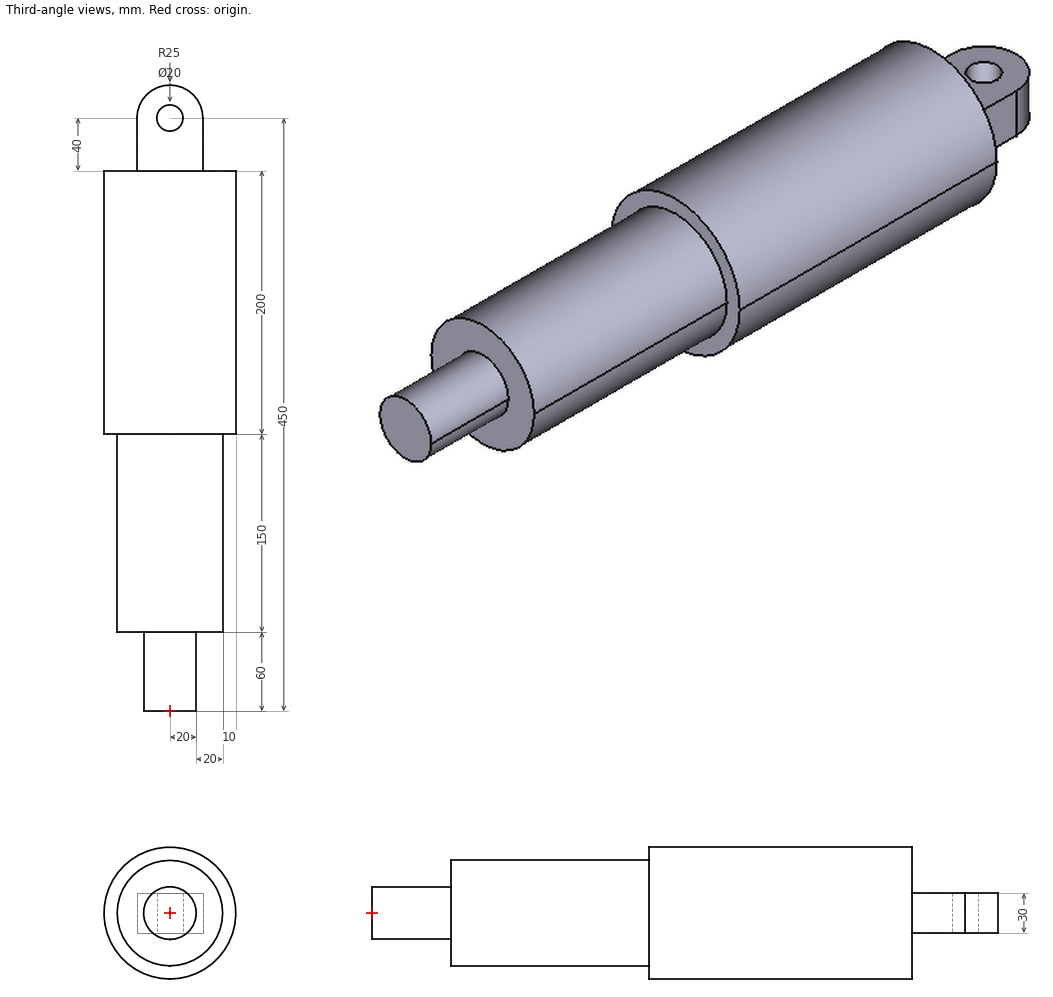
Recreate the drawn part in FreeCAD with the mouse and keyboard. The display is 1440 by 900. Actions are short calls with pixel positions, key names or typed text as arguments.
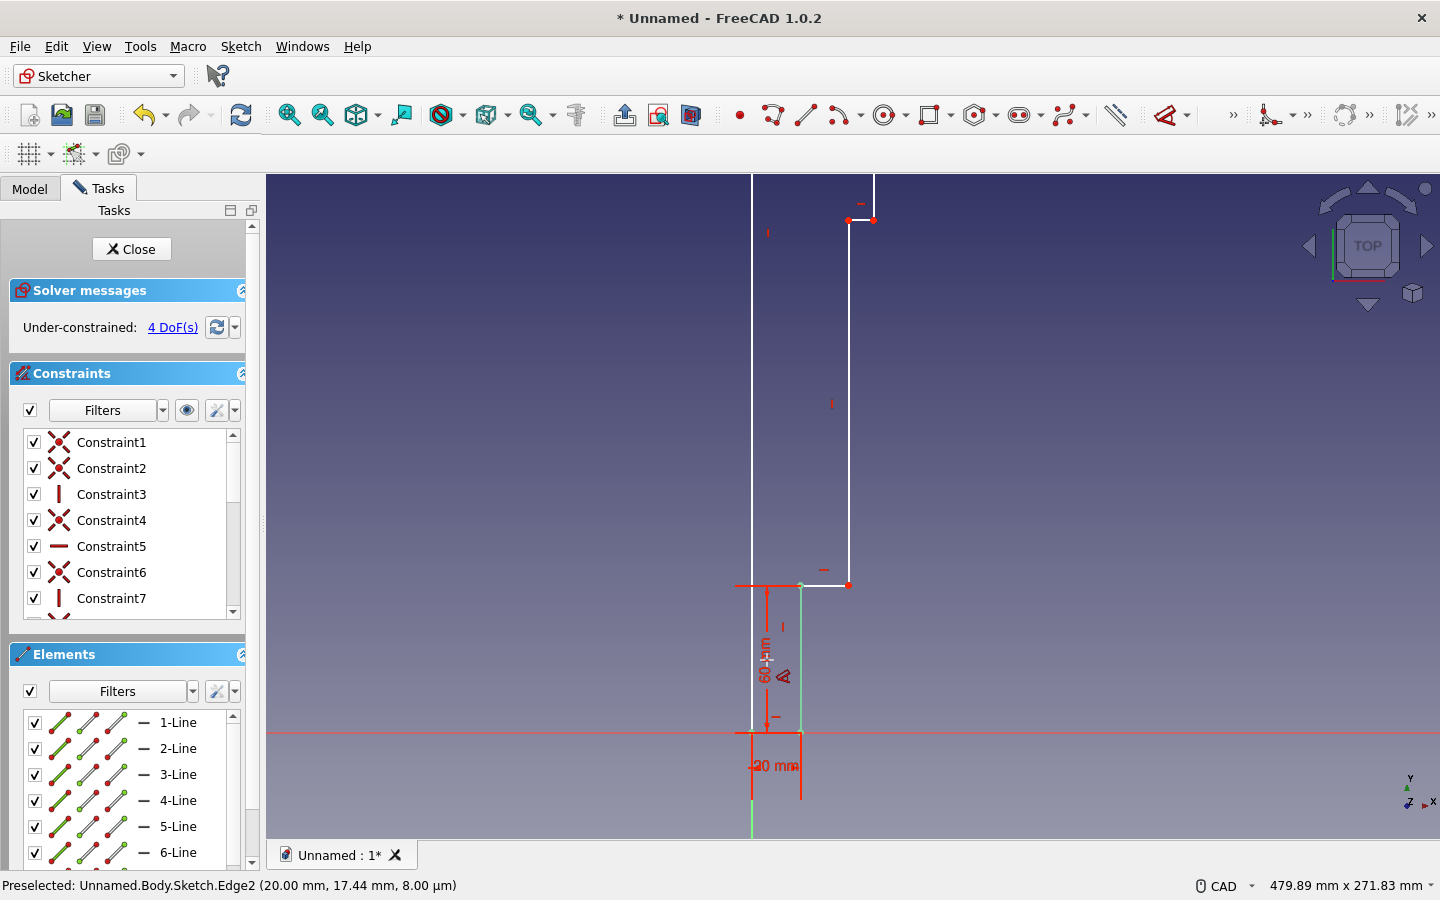
click(815, 586)
click(825, 620)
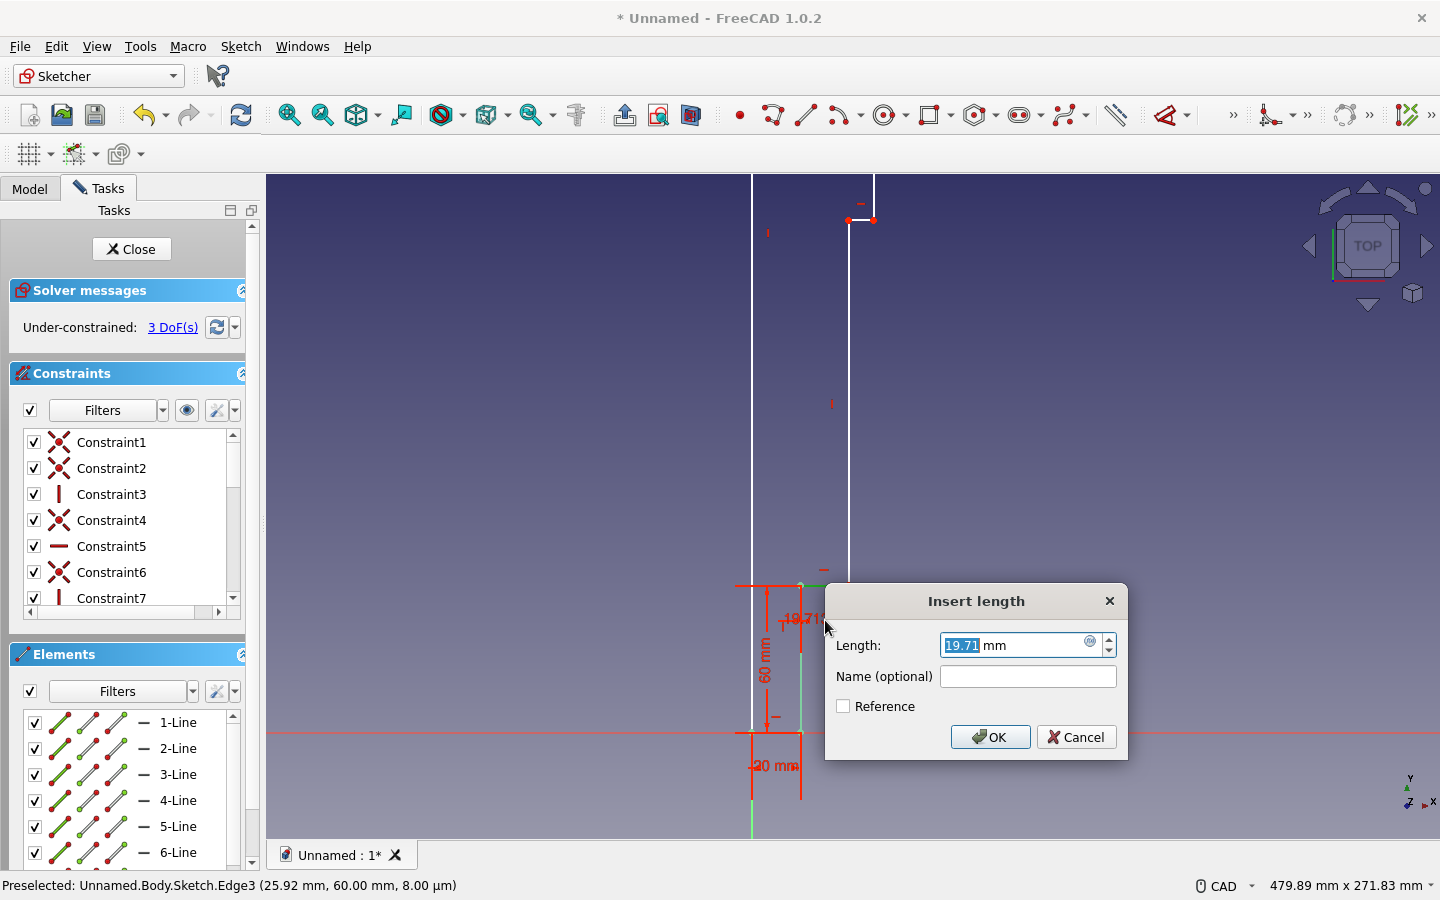
text(20)
key(Return)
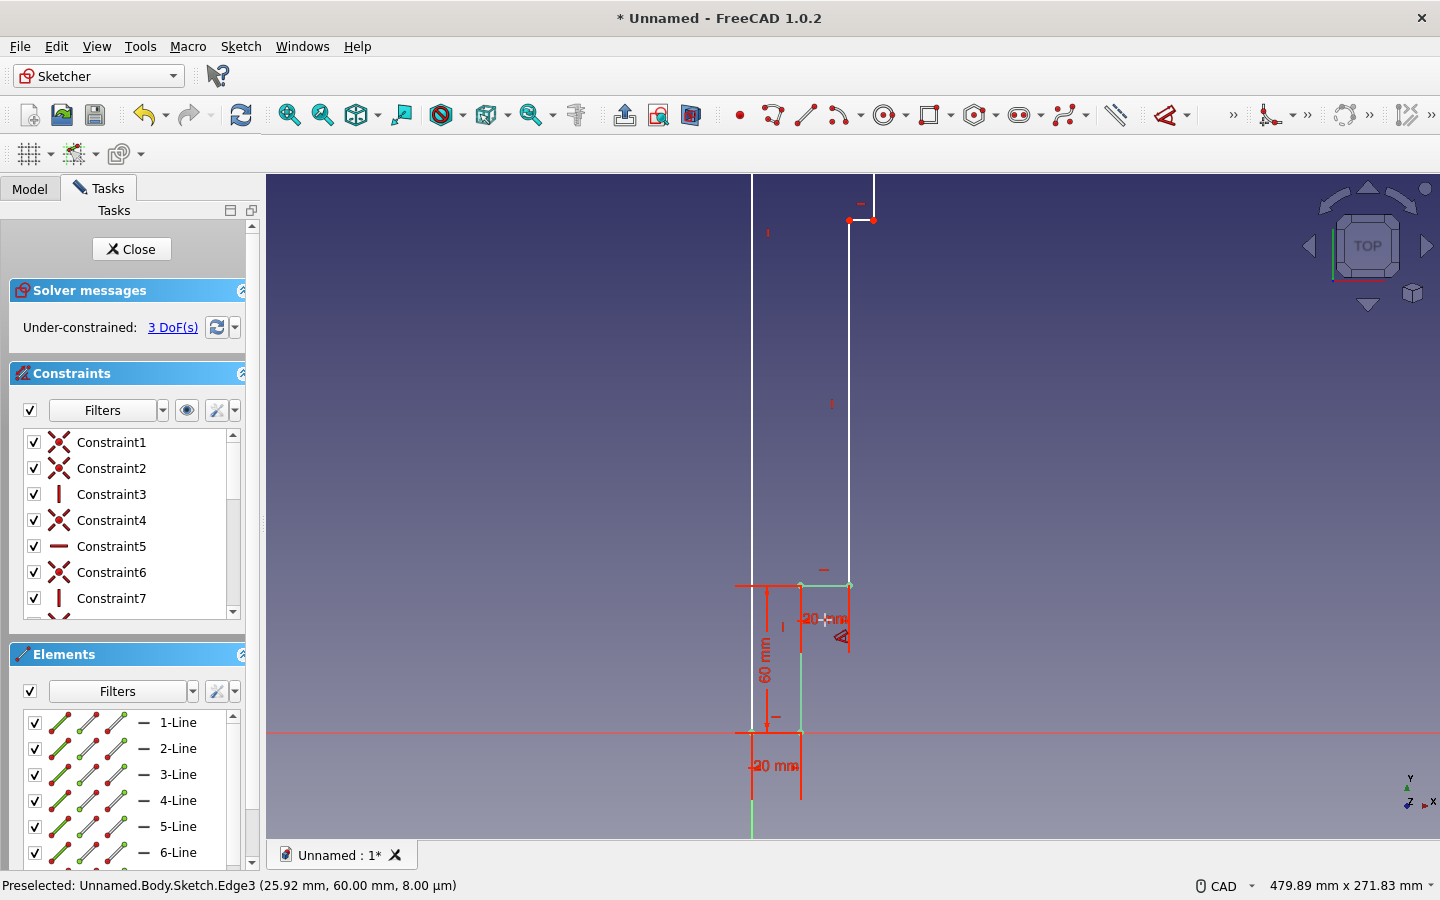
scroll(859, 220, up, 3)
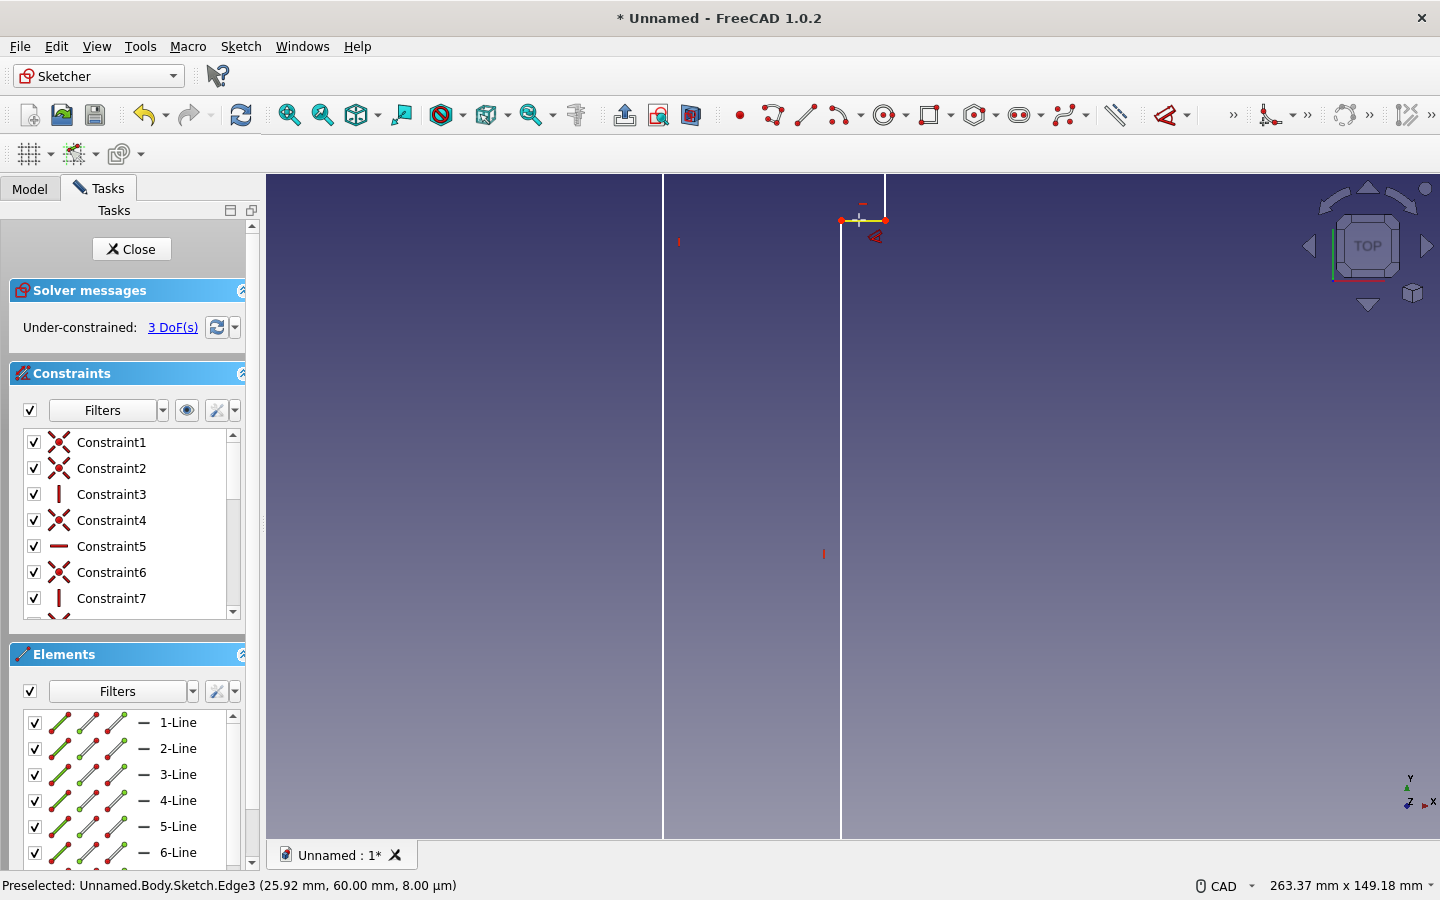
click(859, 221)
click(863, 255)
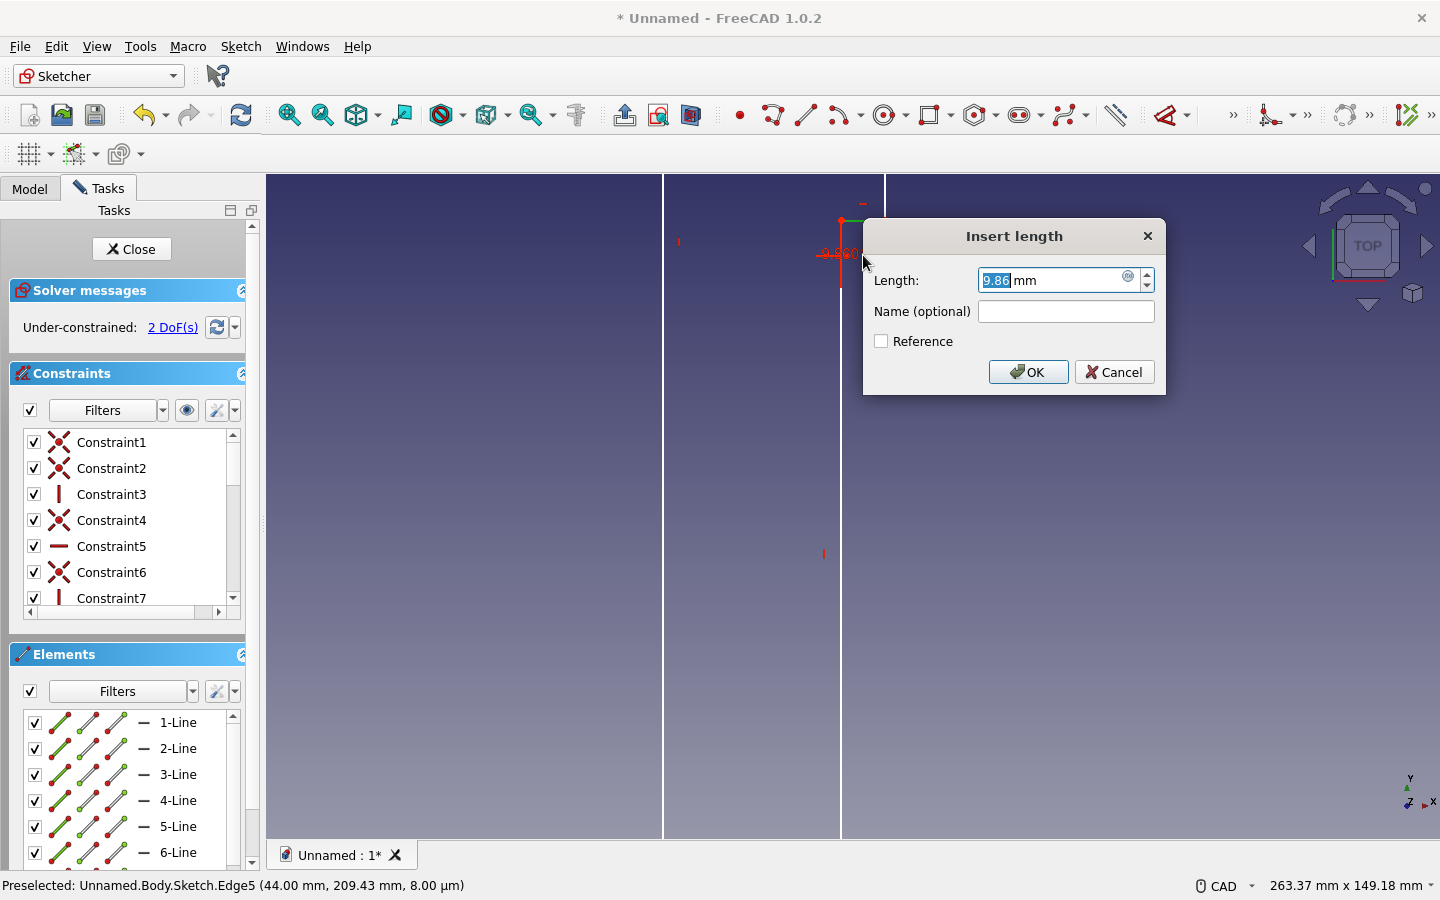
text(10)
key(Return)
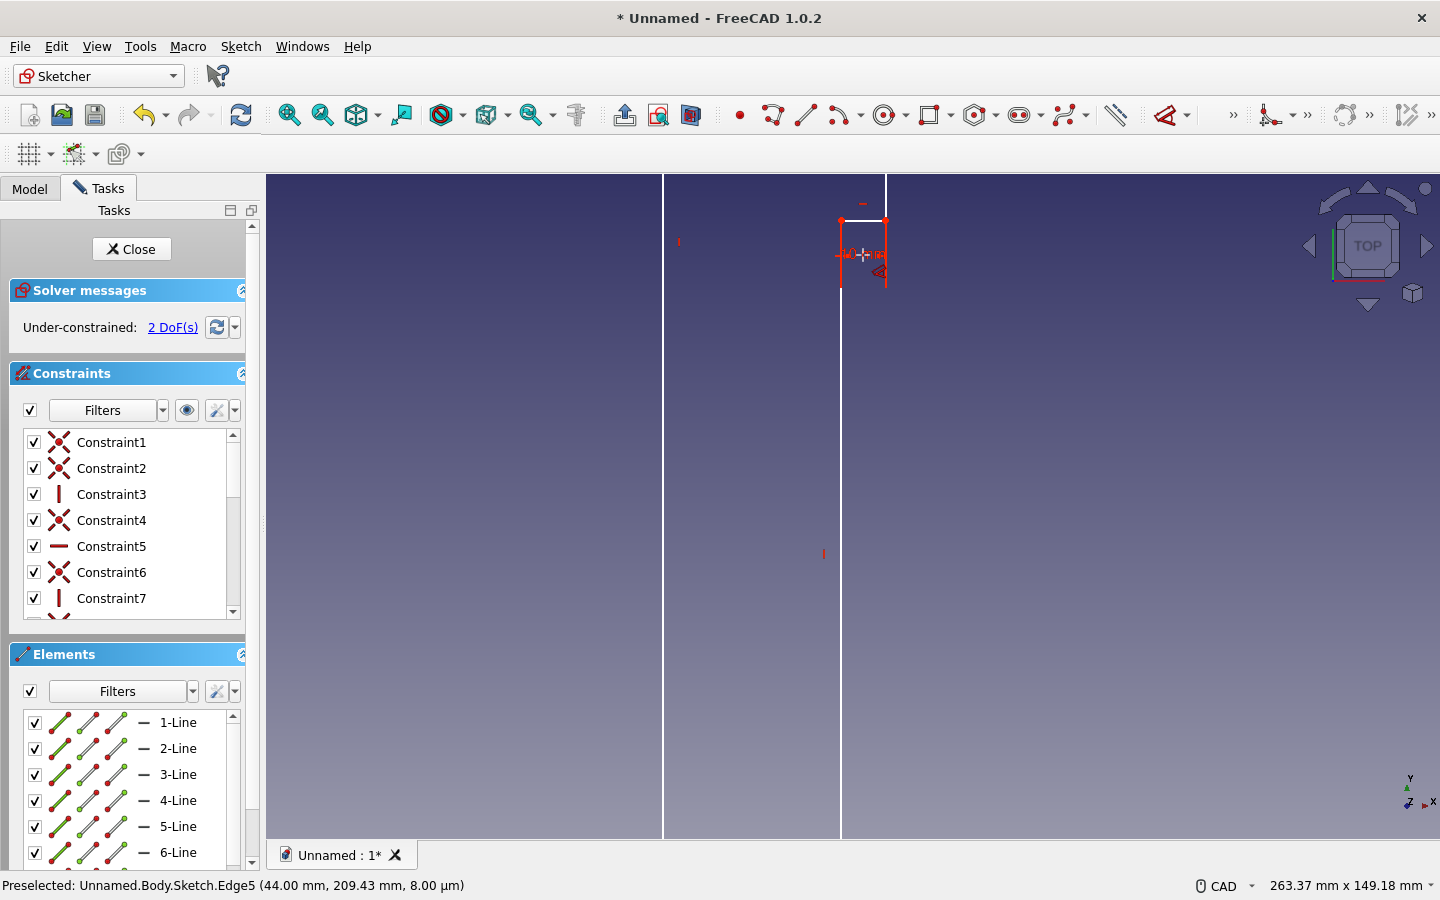
scroll(788, 594, down, 7)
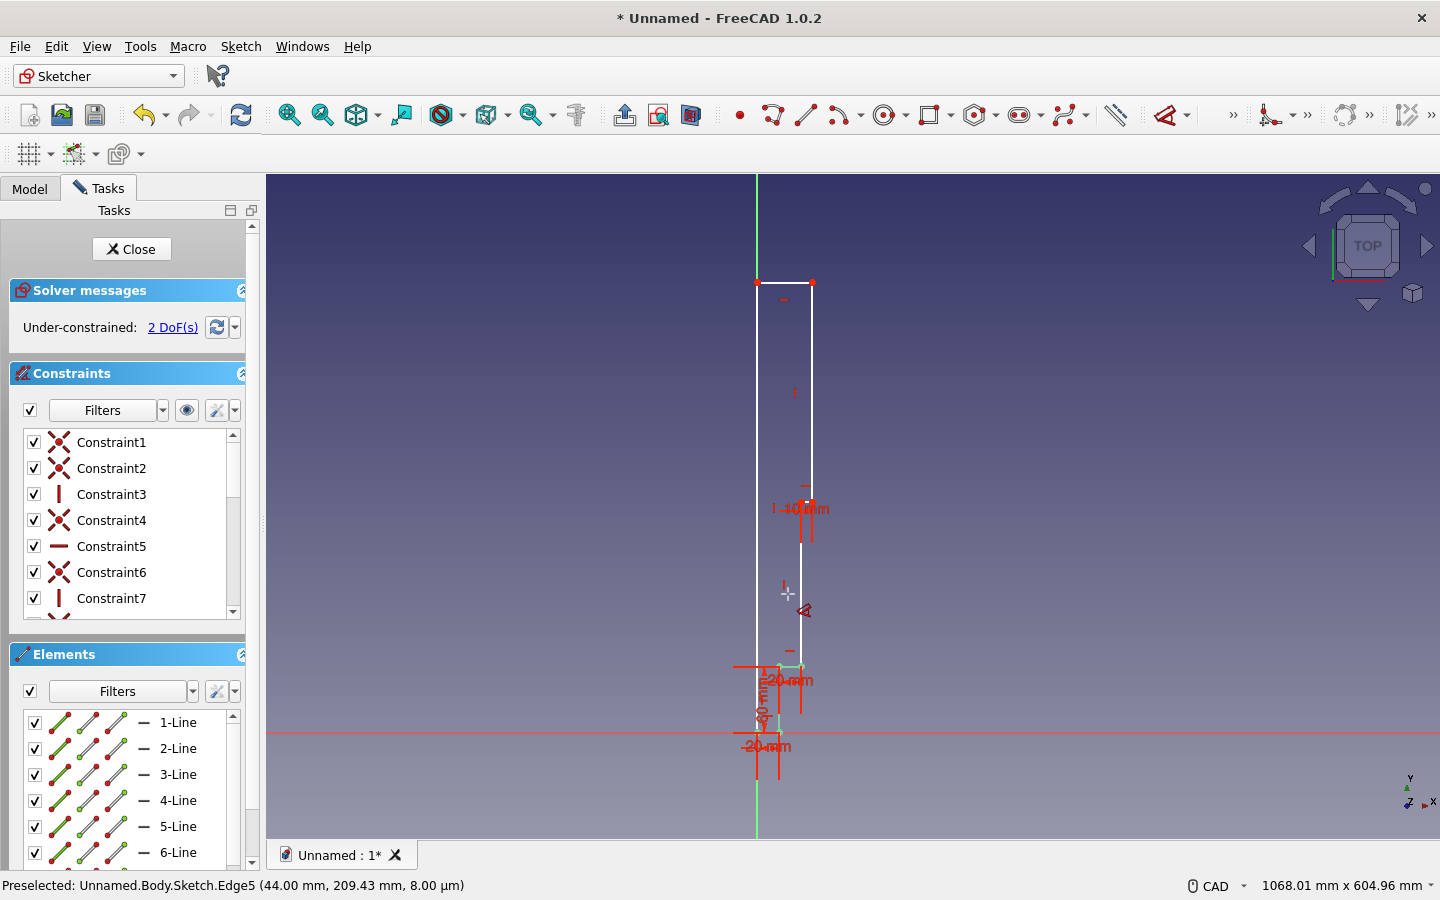
click(801, 617)
click(835, 585)